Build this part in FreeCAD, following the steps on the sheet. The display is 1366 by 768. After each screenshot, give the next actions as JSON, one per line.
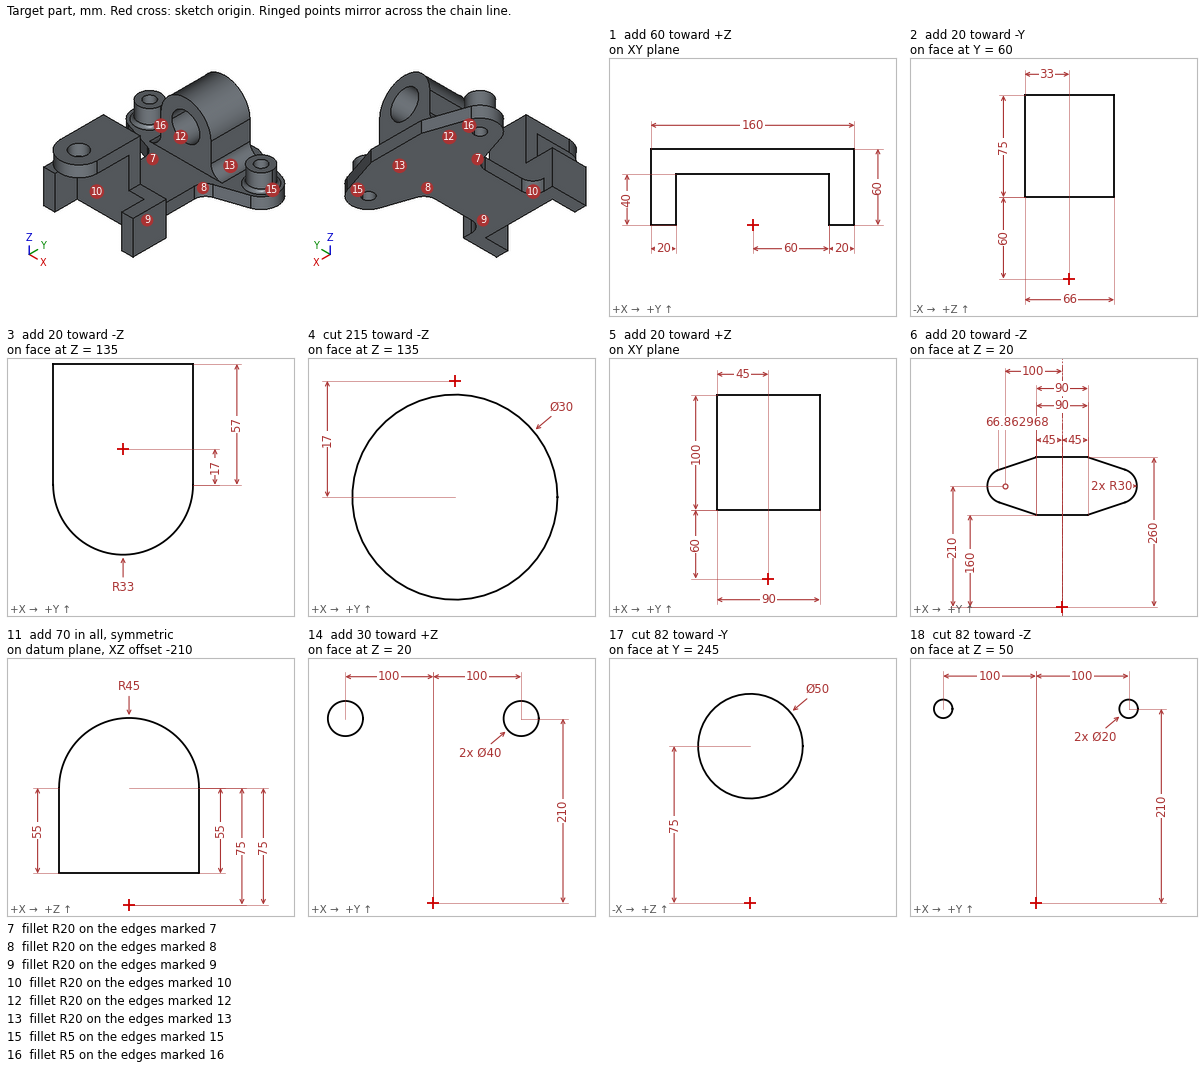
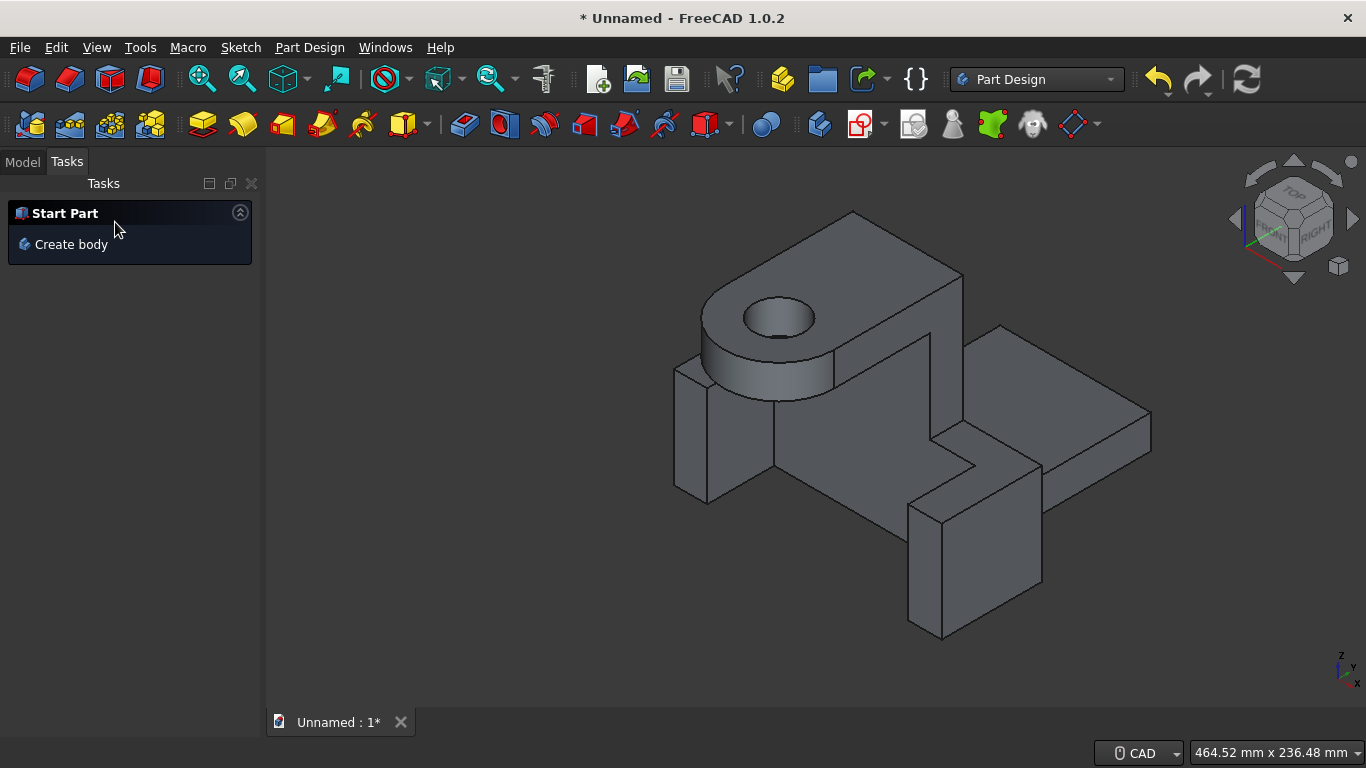
{"action": "key", "text": "v f"}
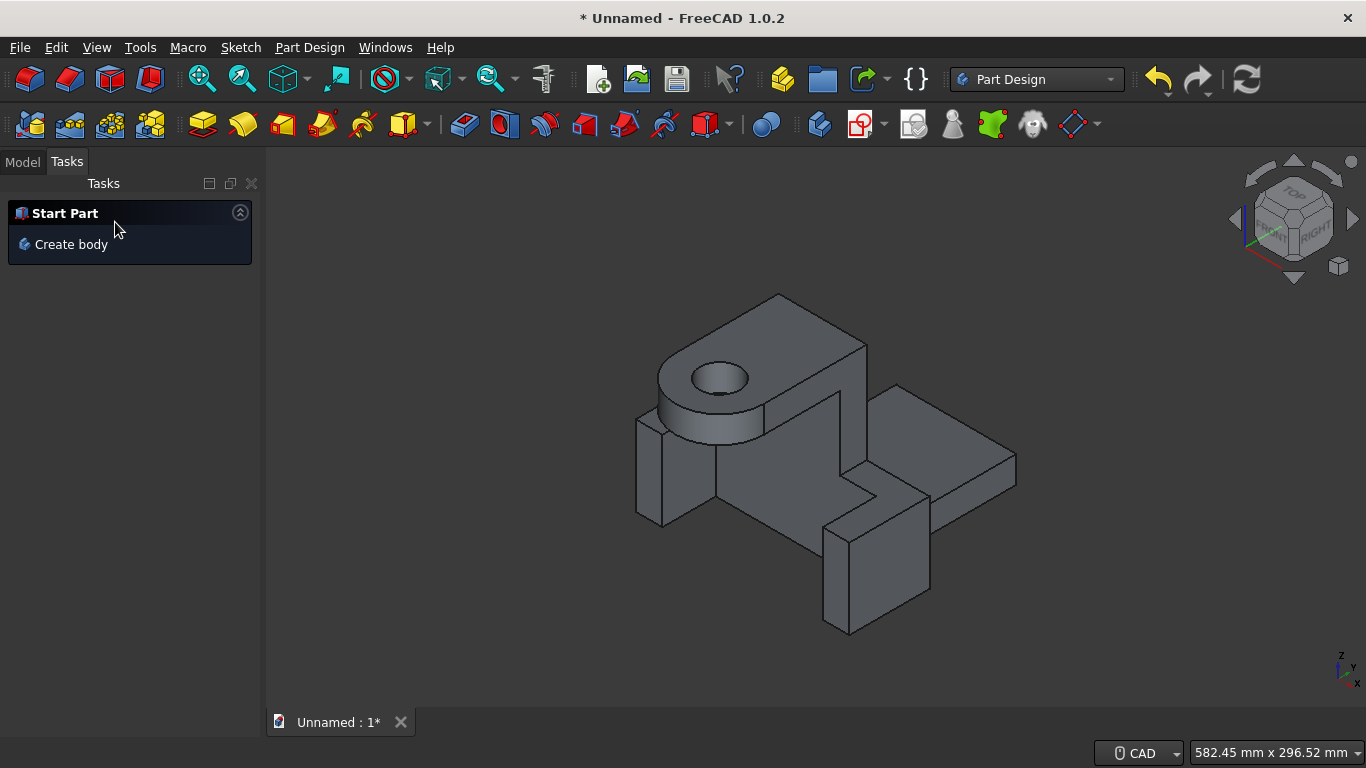
{"action": "left_click", "coordinate": [889, 457]}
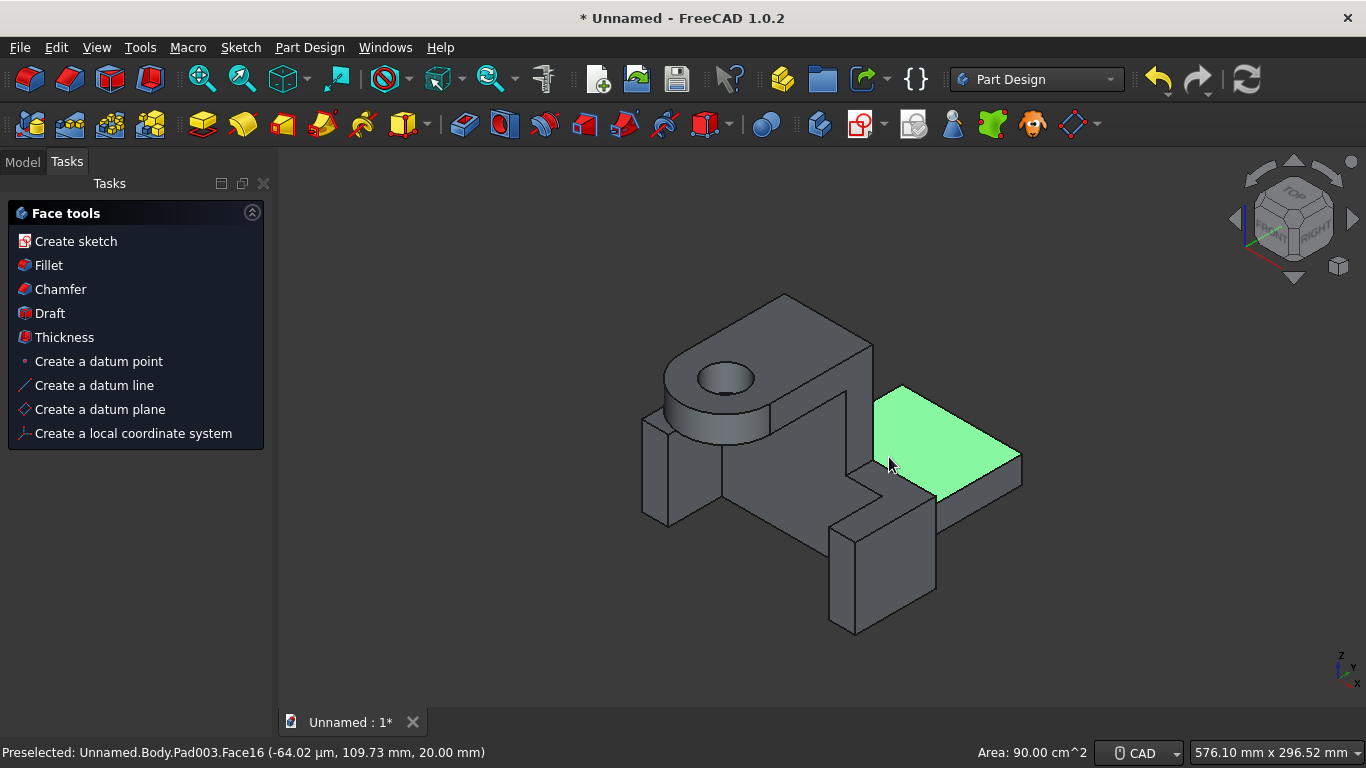
{"action": "left_click", "coordinate": [860, 124]}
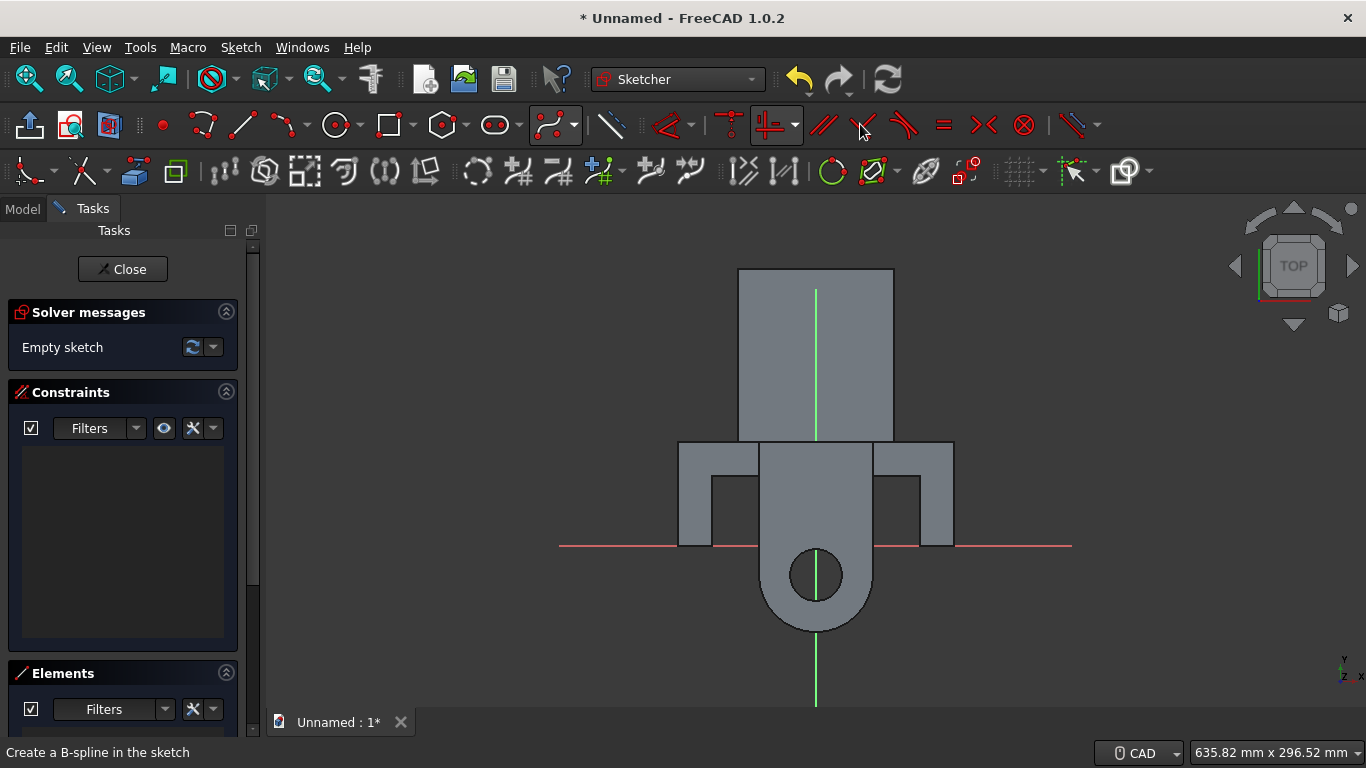
{"action": "key", "text": "q s"}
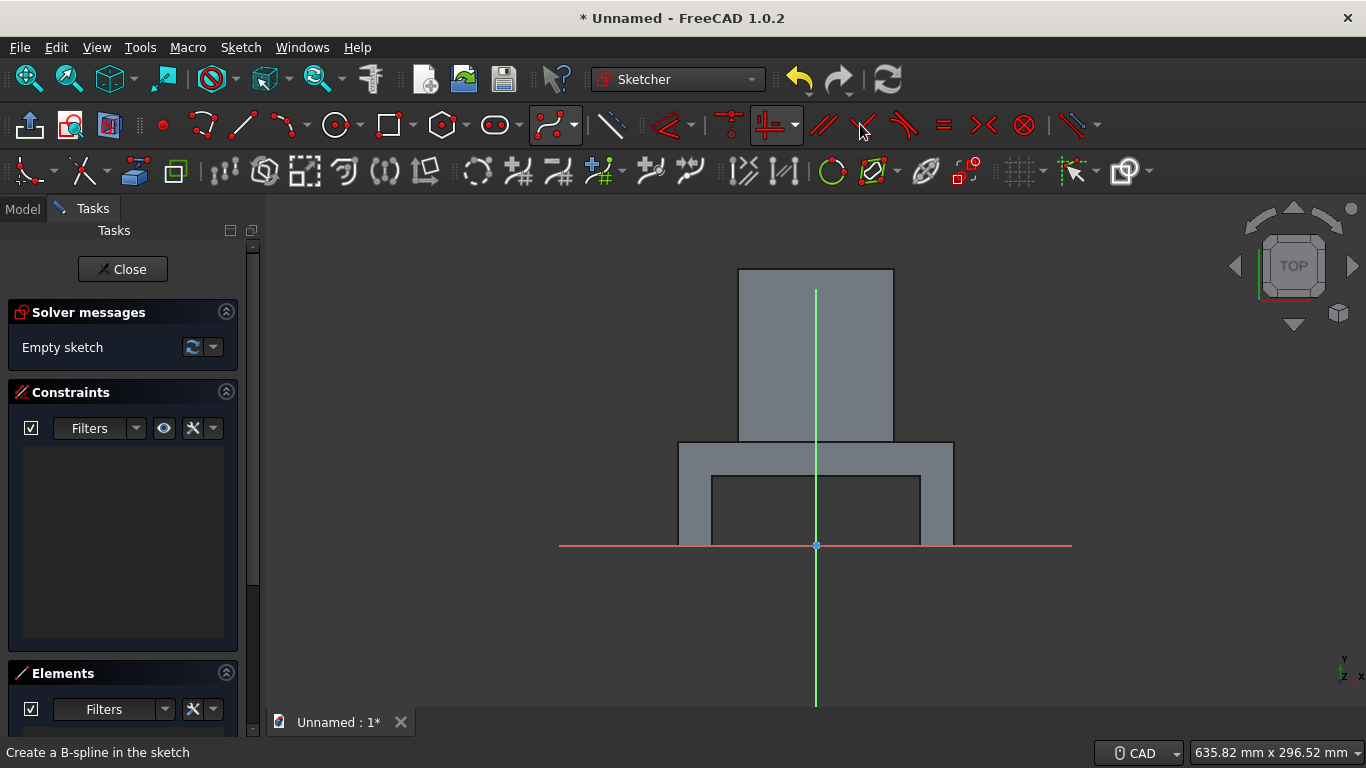
{"action": "scroll", "coordinate": [608, 679], "scroll_direction": "down", "scroll_amount": 2}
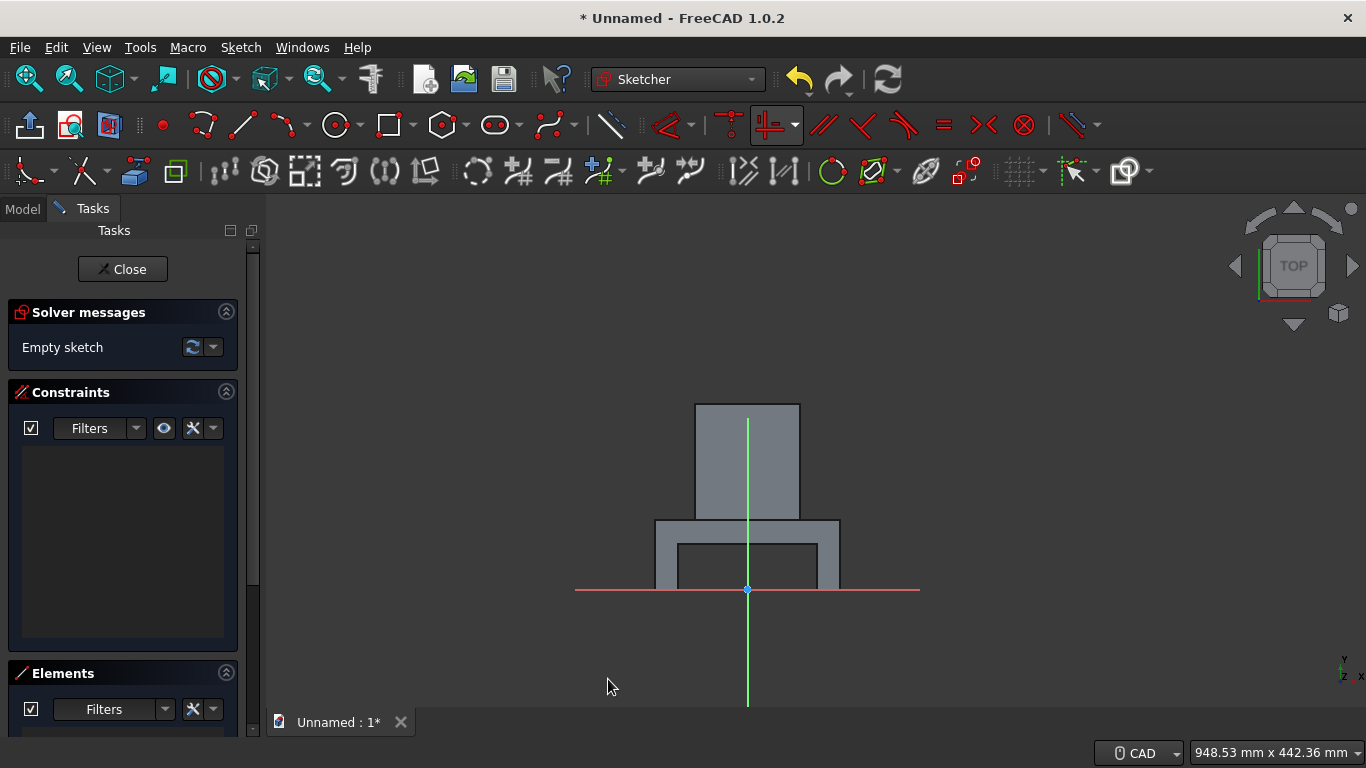
{"action": "key", "text": "g m"}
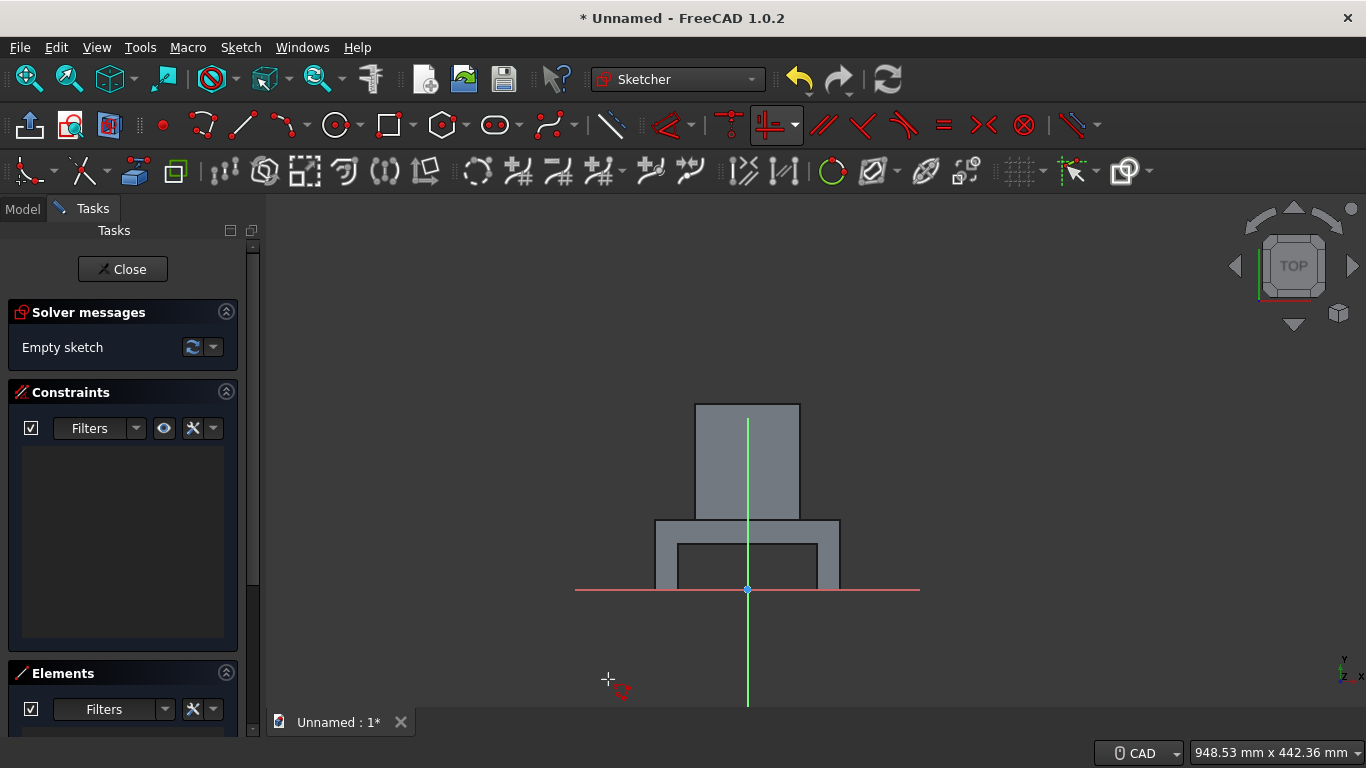
{"action": "left_click", "coordinate": [875, 313]}
{"action": "left_click", "coordinate": [800, 288]}
{"action": "left_click", "coordinate": [695, 288]}
{"action": "left_click", "coordinate": [618, 314]}
{"action": "right_click", "coordinate": [618, 314]}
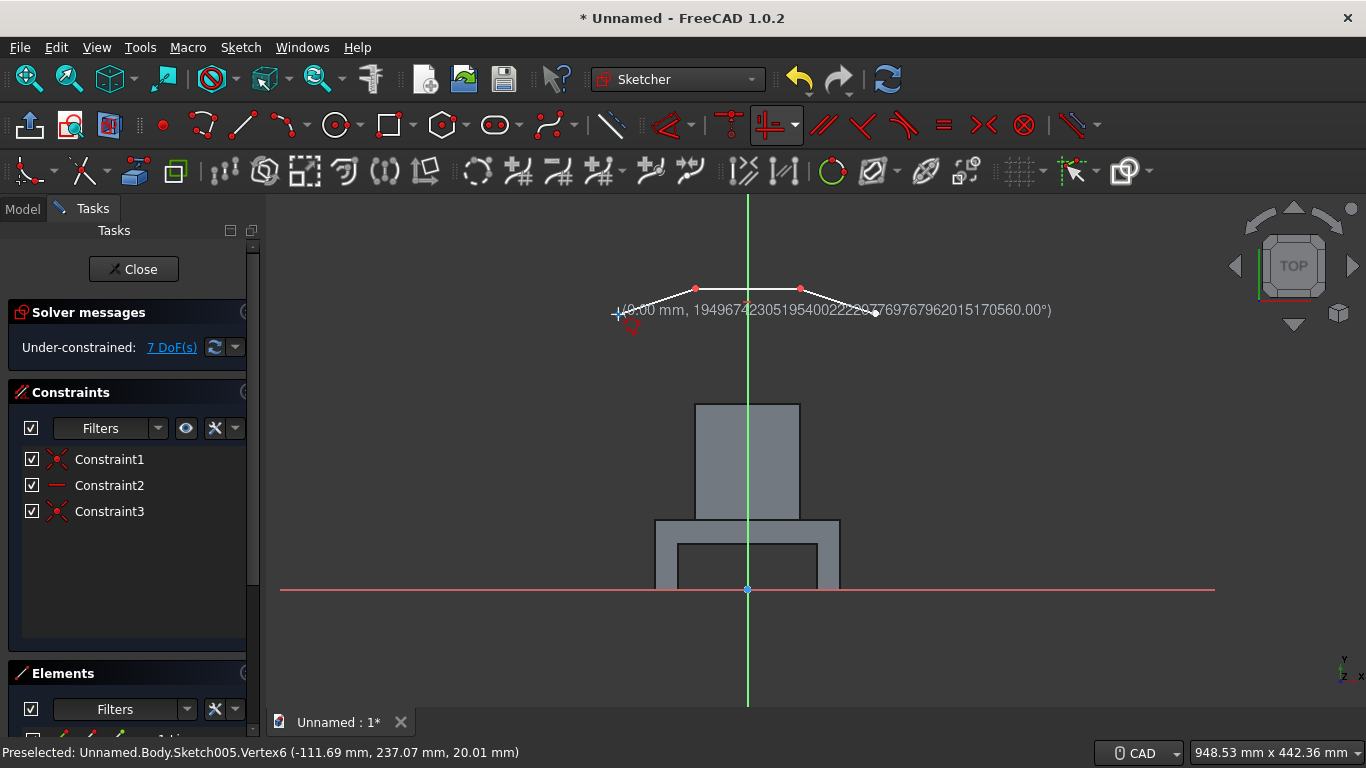
{"action": "left_click", "coordinate": [621, 379]}
{"action": "left_click", "coordinate": [695, 404]}
{"action": "left_click", "coordinate": [800, 404]}
{"action": "left_click", "coordinate": [875, 379]}
{"action": "right_click", "coordinate": [875, 379]}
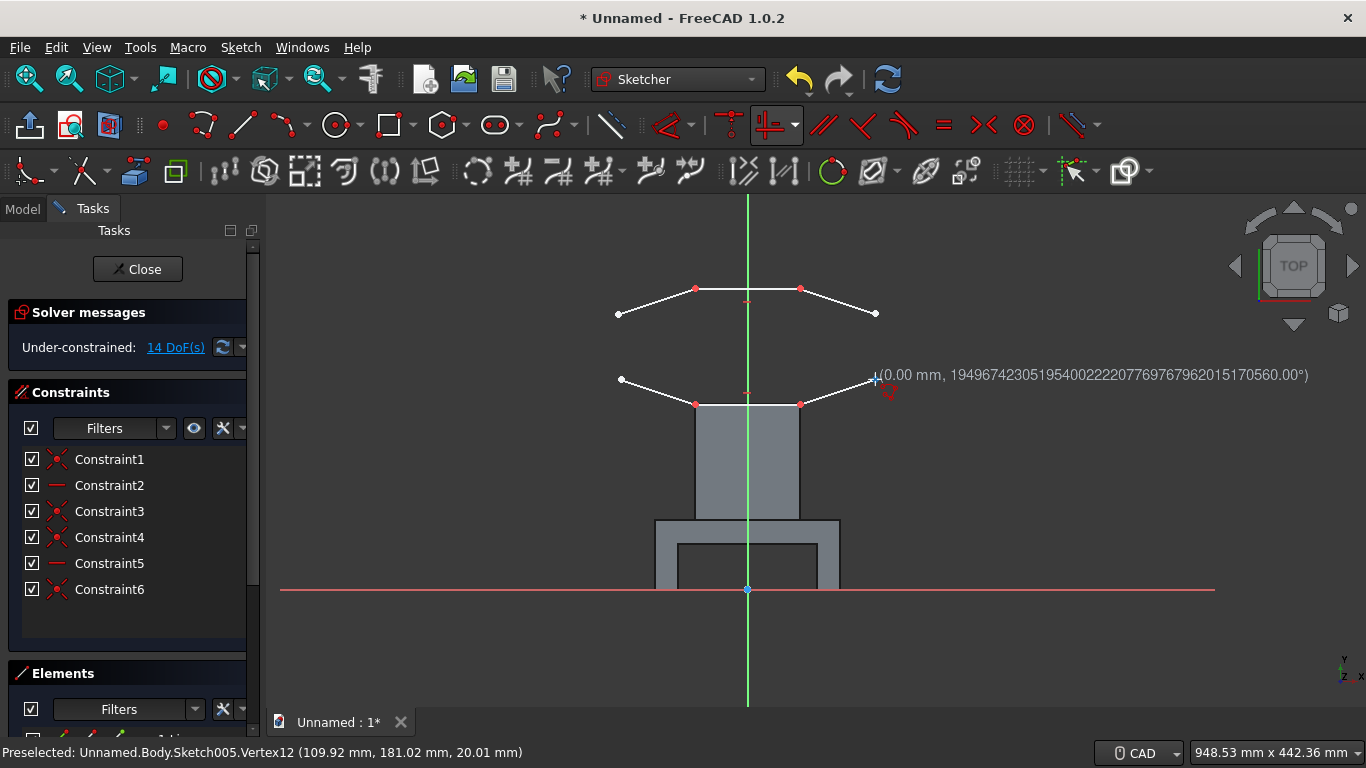
{"action": "left_click", "coordinate": [284, 126]}